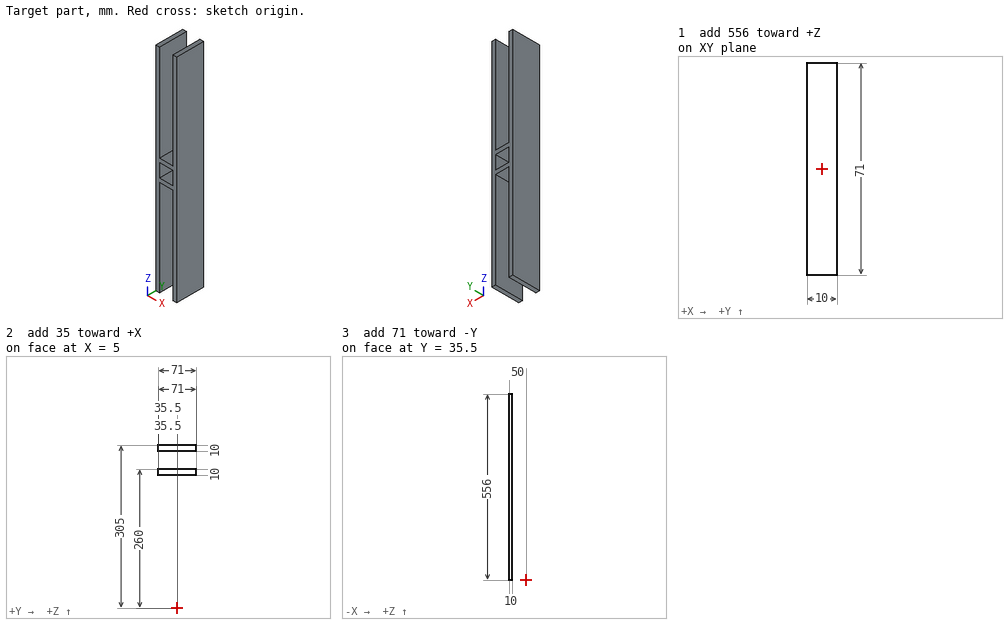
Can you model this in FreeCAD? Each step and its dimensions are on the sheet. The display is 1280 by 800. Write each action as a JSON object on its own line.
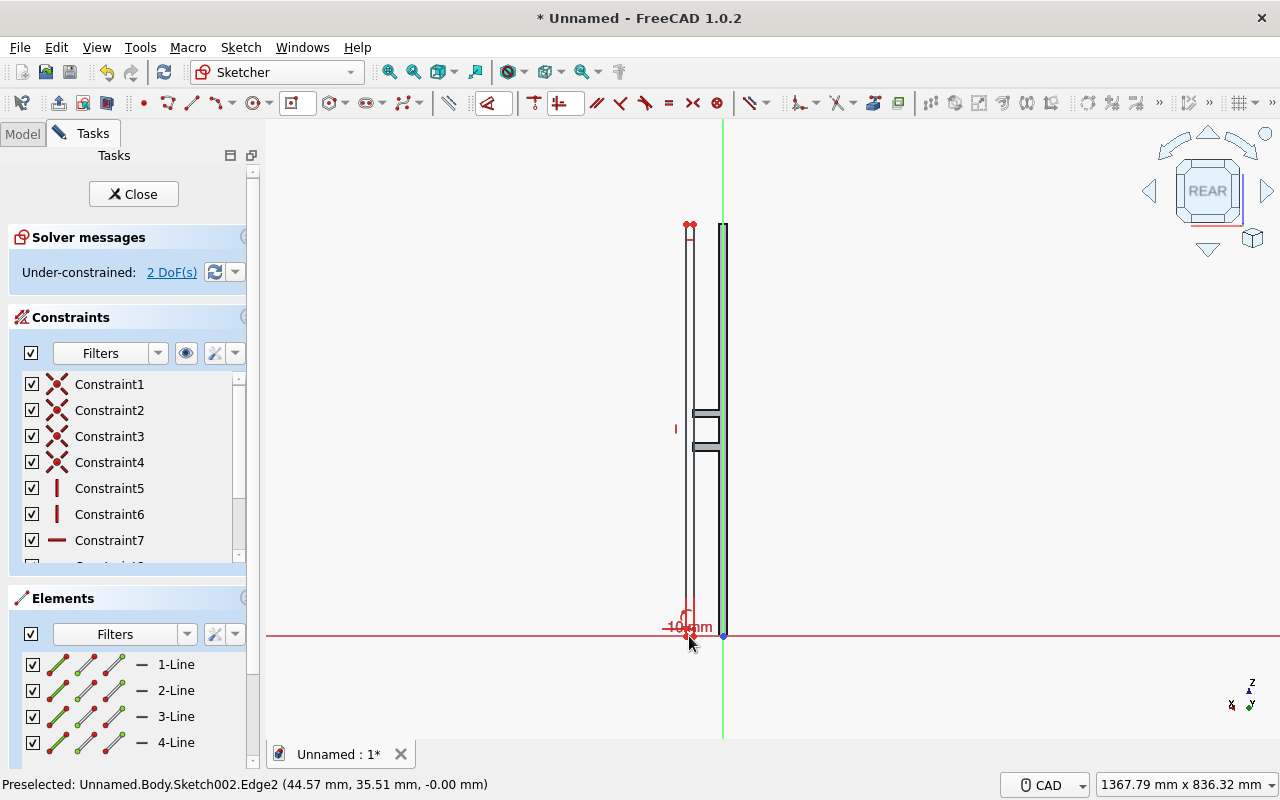
{"action": "scroll", "coordinate": [686, 348], "scroll_direction": "up", "scroll_amount": 4}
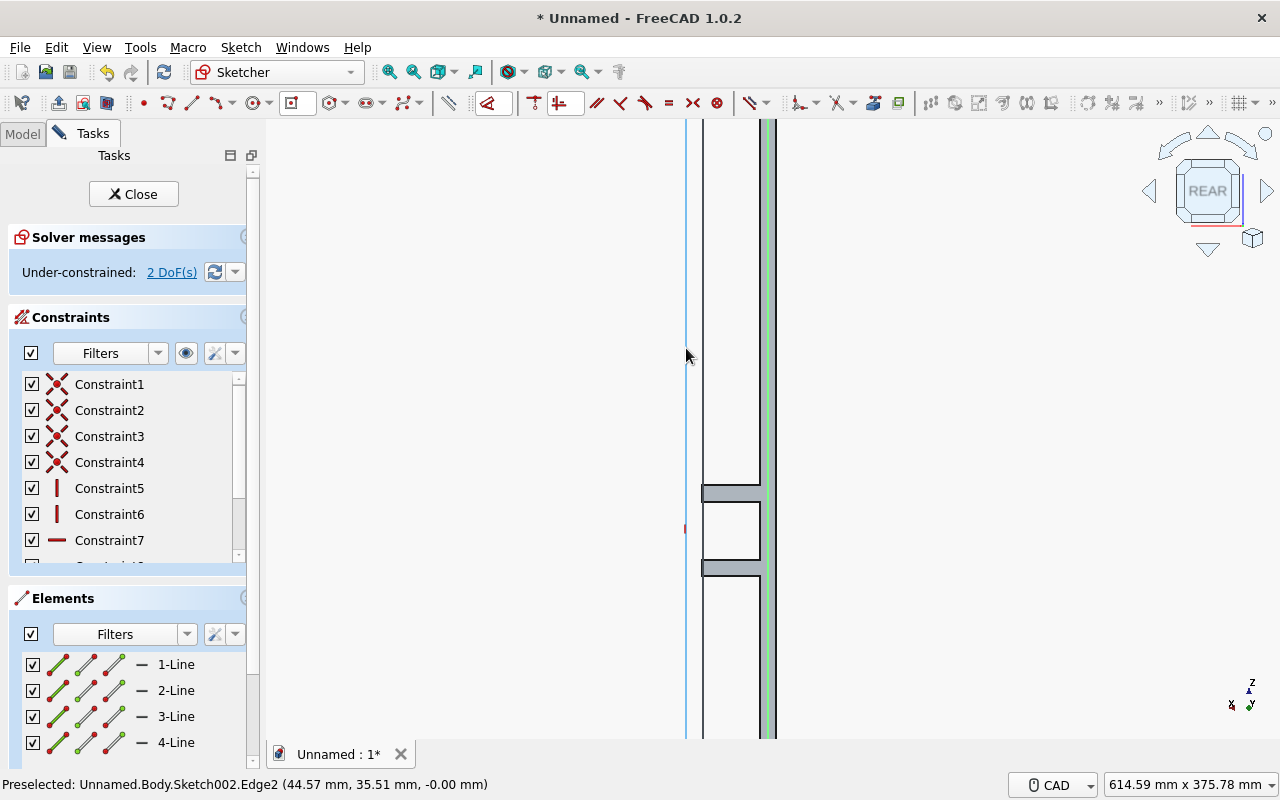
{"action": "left_click", "coordinate": [686, 347]}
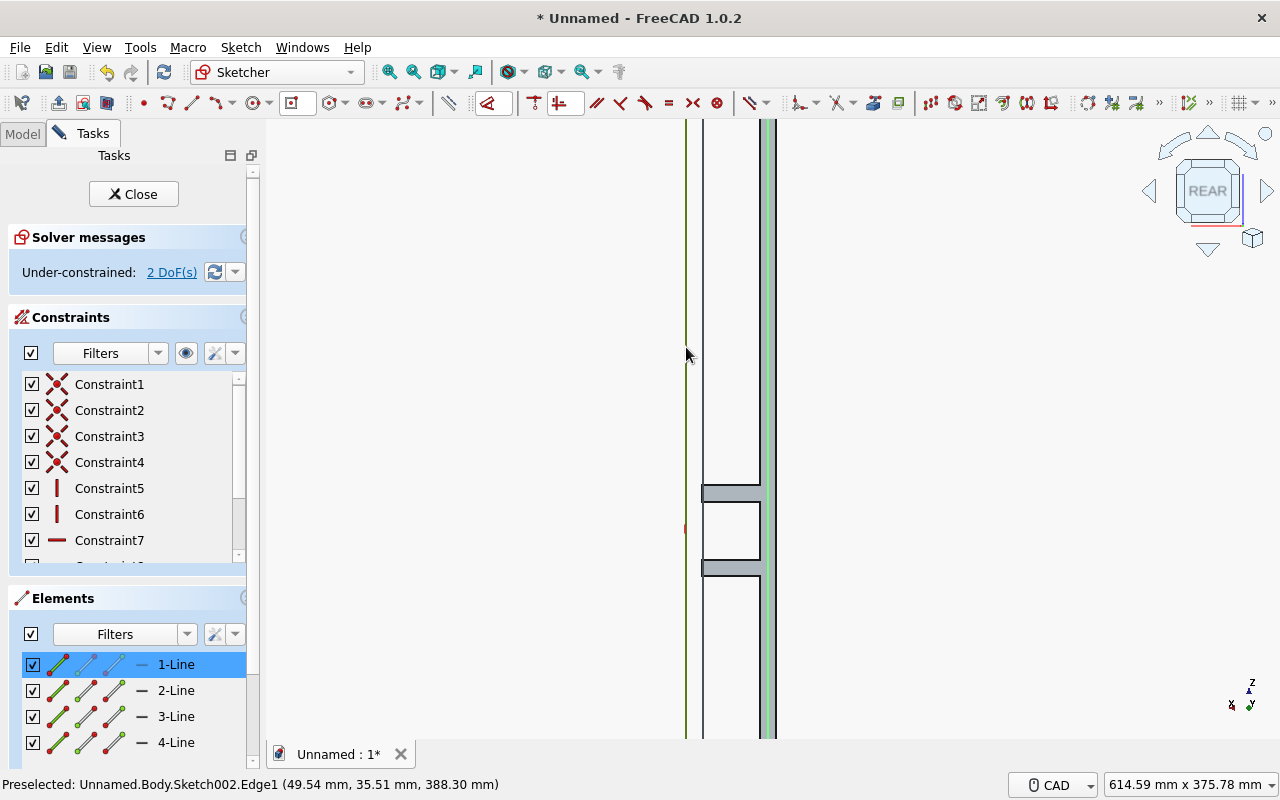
{"action": "key", "text": "i"}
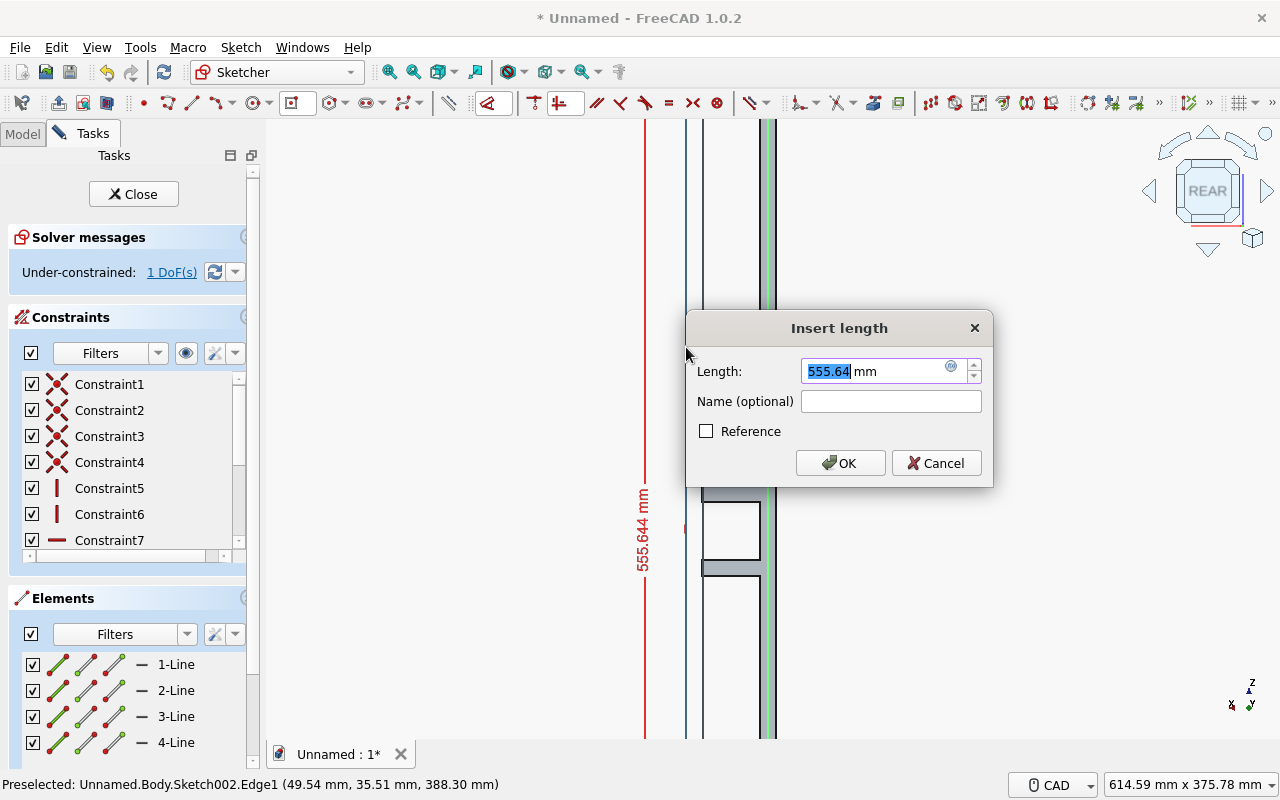
{"action": "type", "text": "556"}
{"action": "key", "text": "Return"}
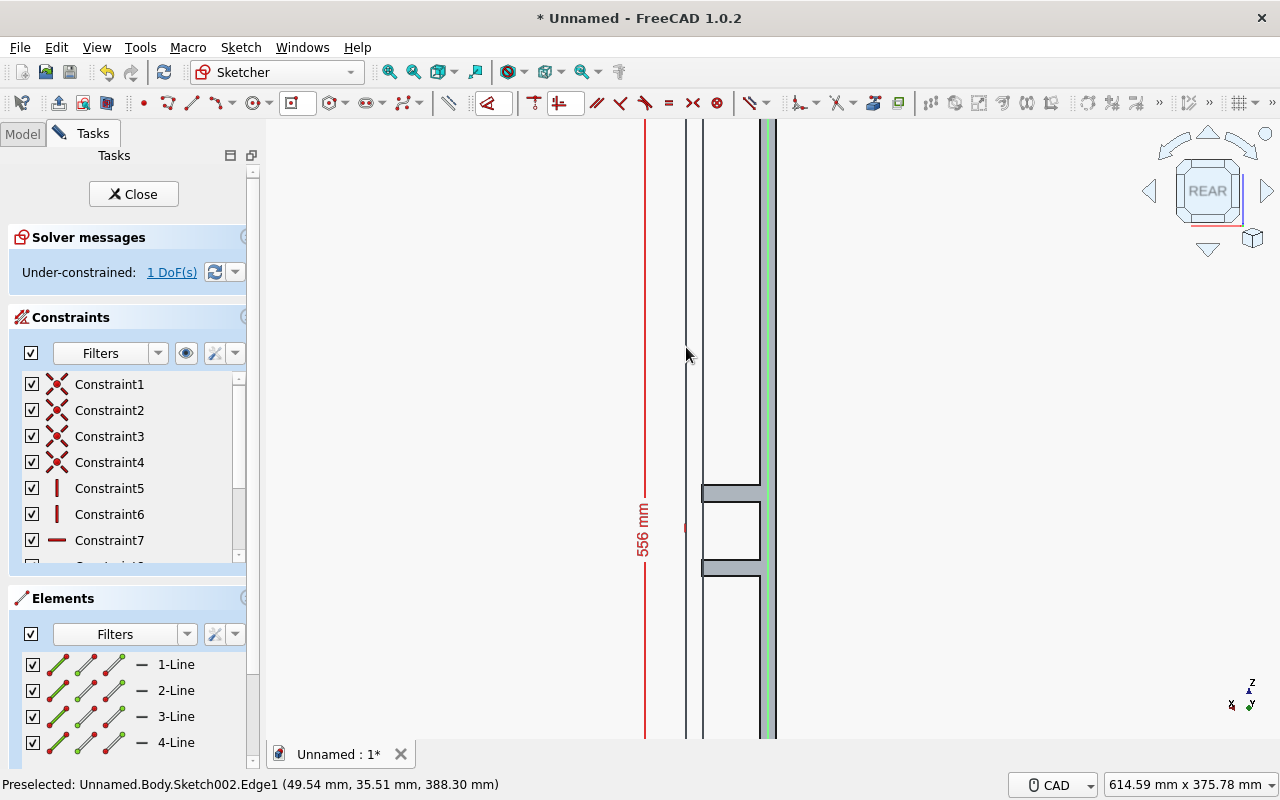
{"action": "scroll", "coordinate": [686, 347], "scroll_direction": "down", "scroll_amount": 4}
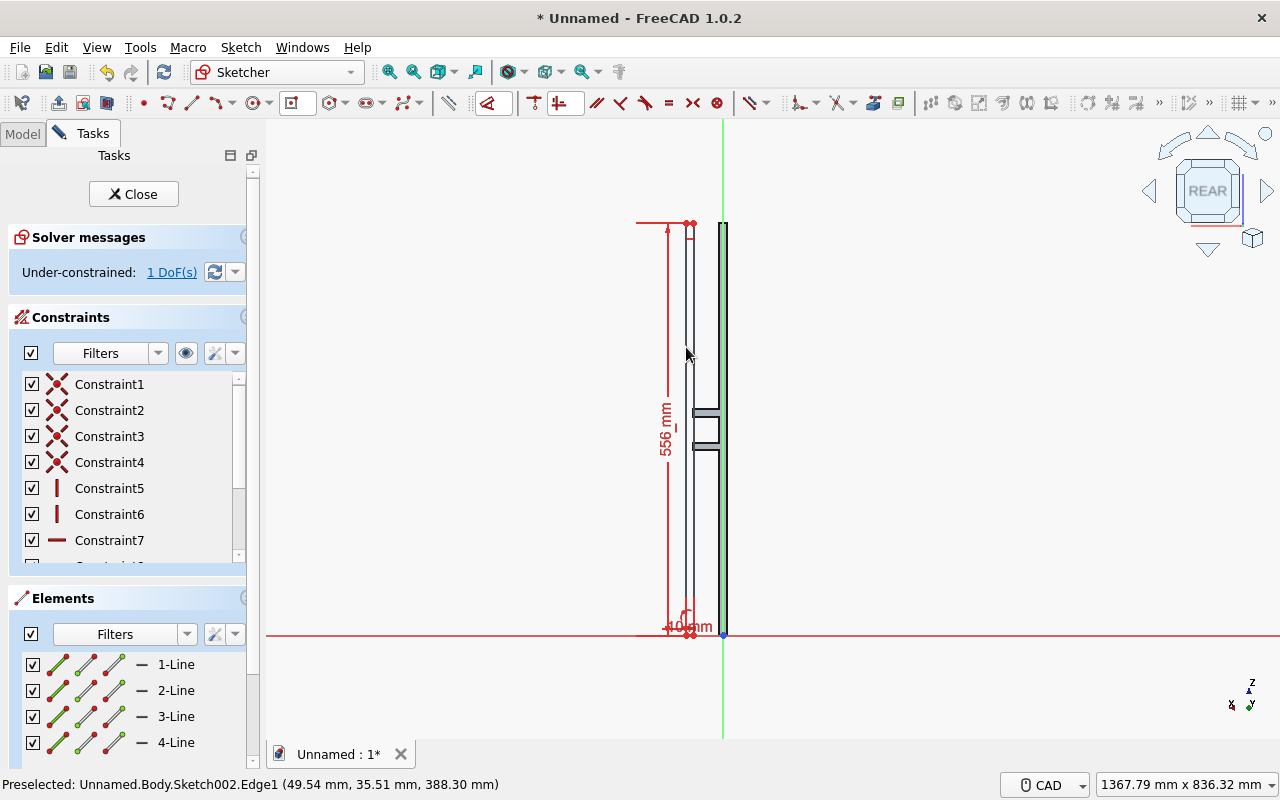
{"action": "scroll", "coordinate": [686, 223], "scroll_direction": "up", "scroll_amount": 3}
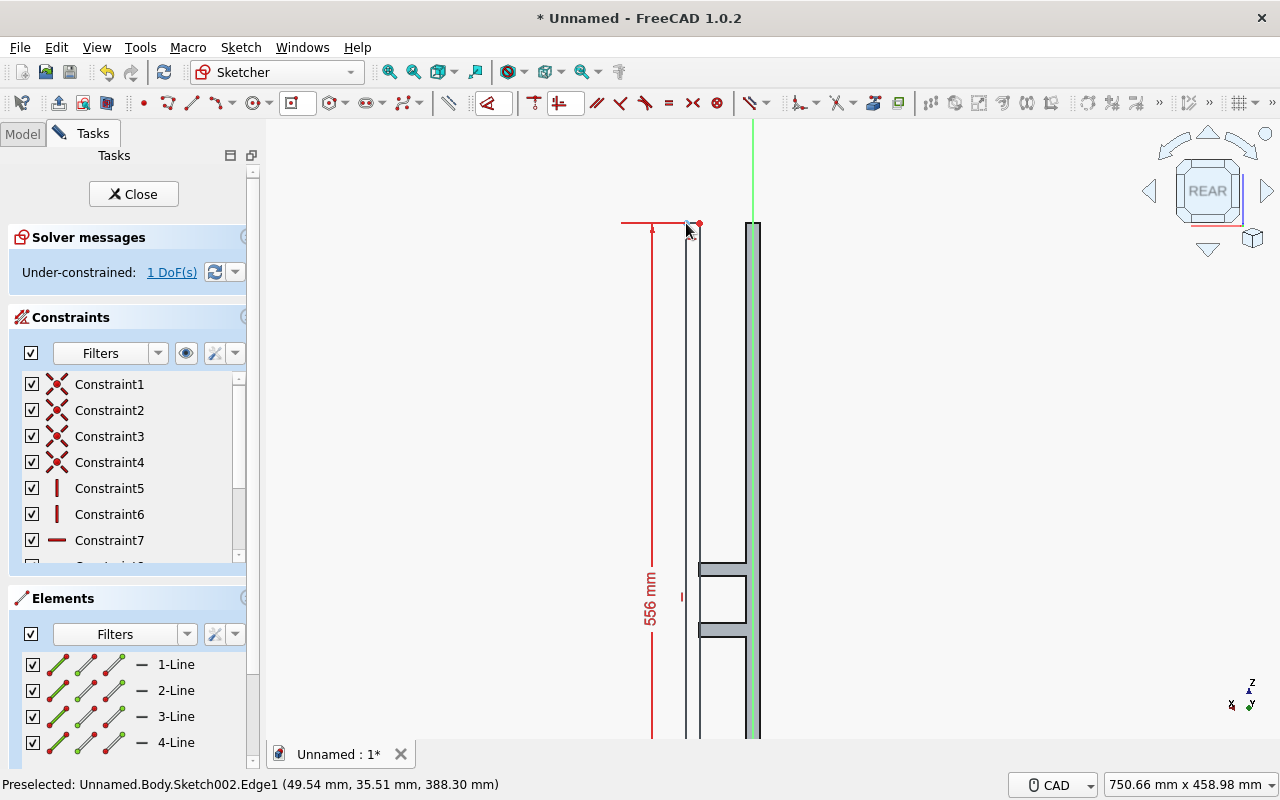
{"action": "left_click", "coordinate": [686, 223]}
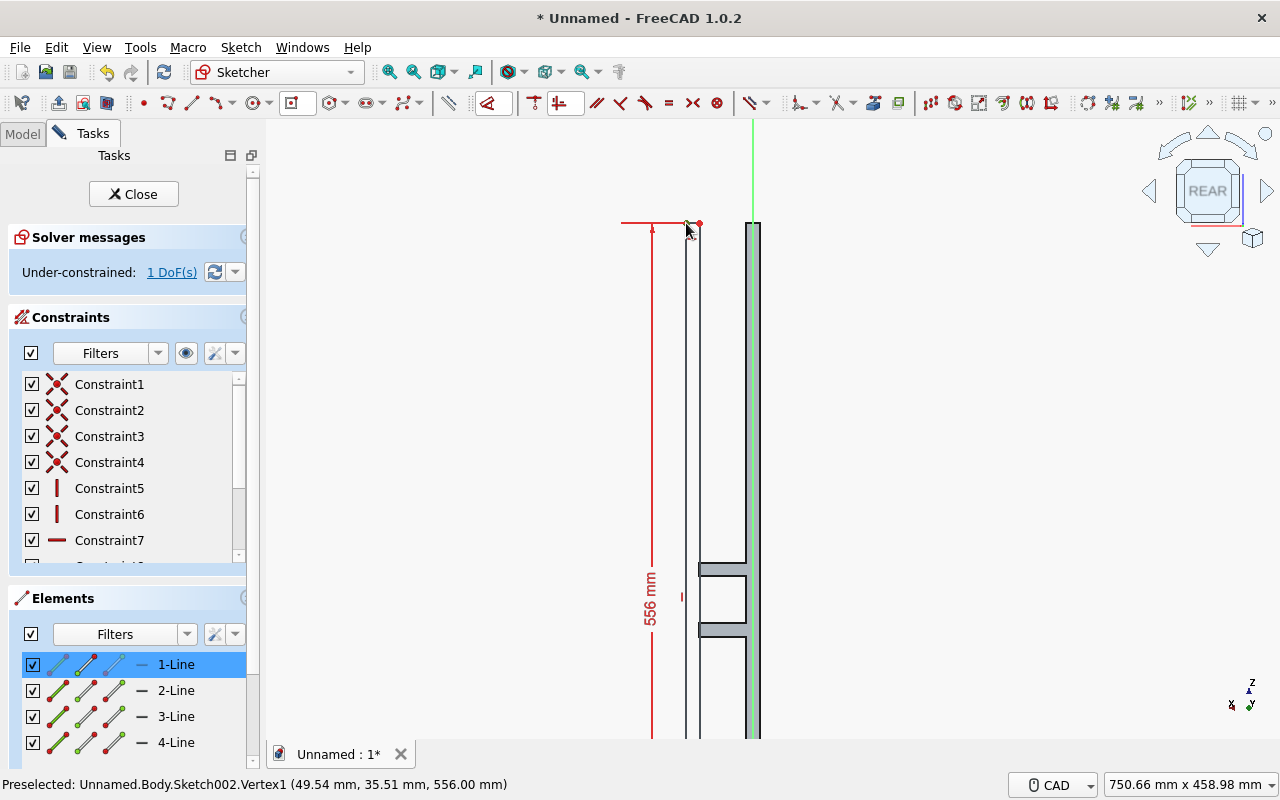
{"action": "key", "text": "l"}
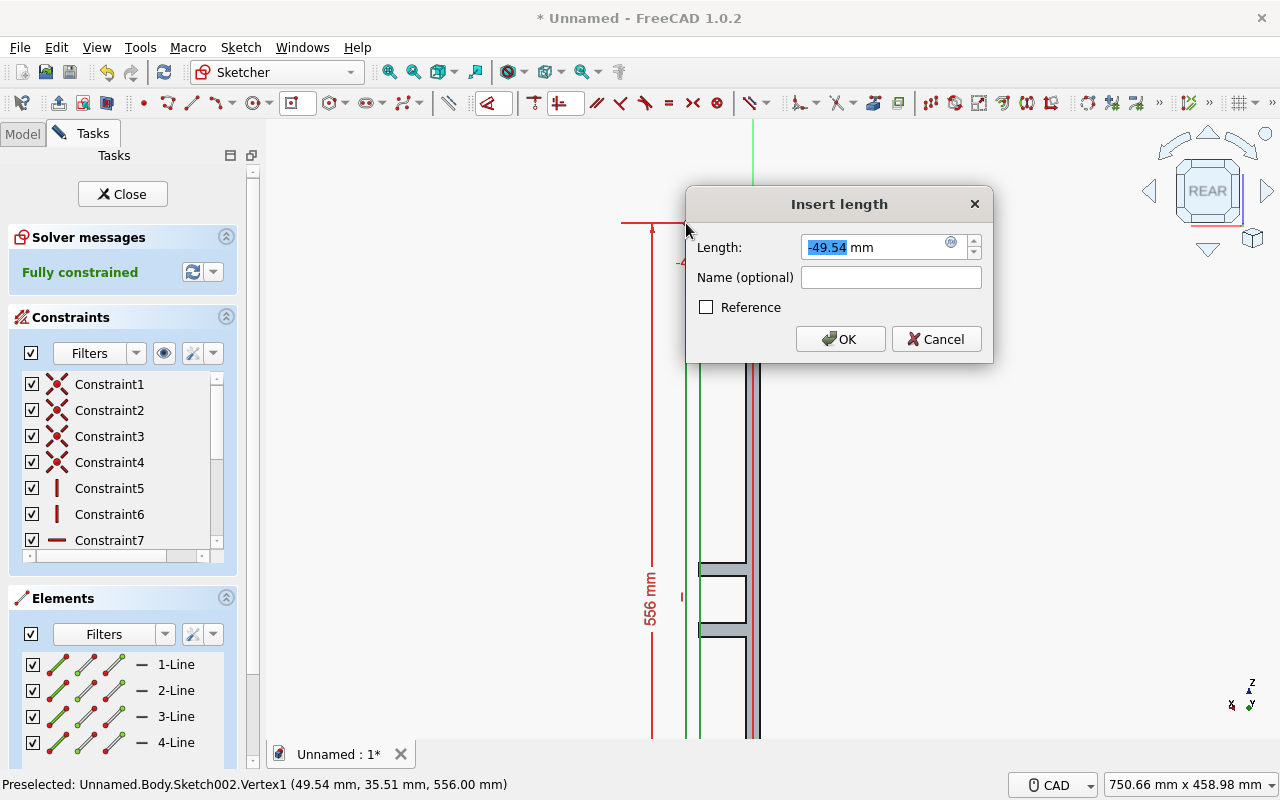
{"action": "type", "text": "-50"}
{"action": "key", "text": "Return"}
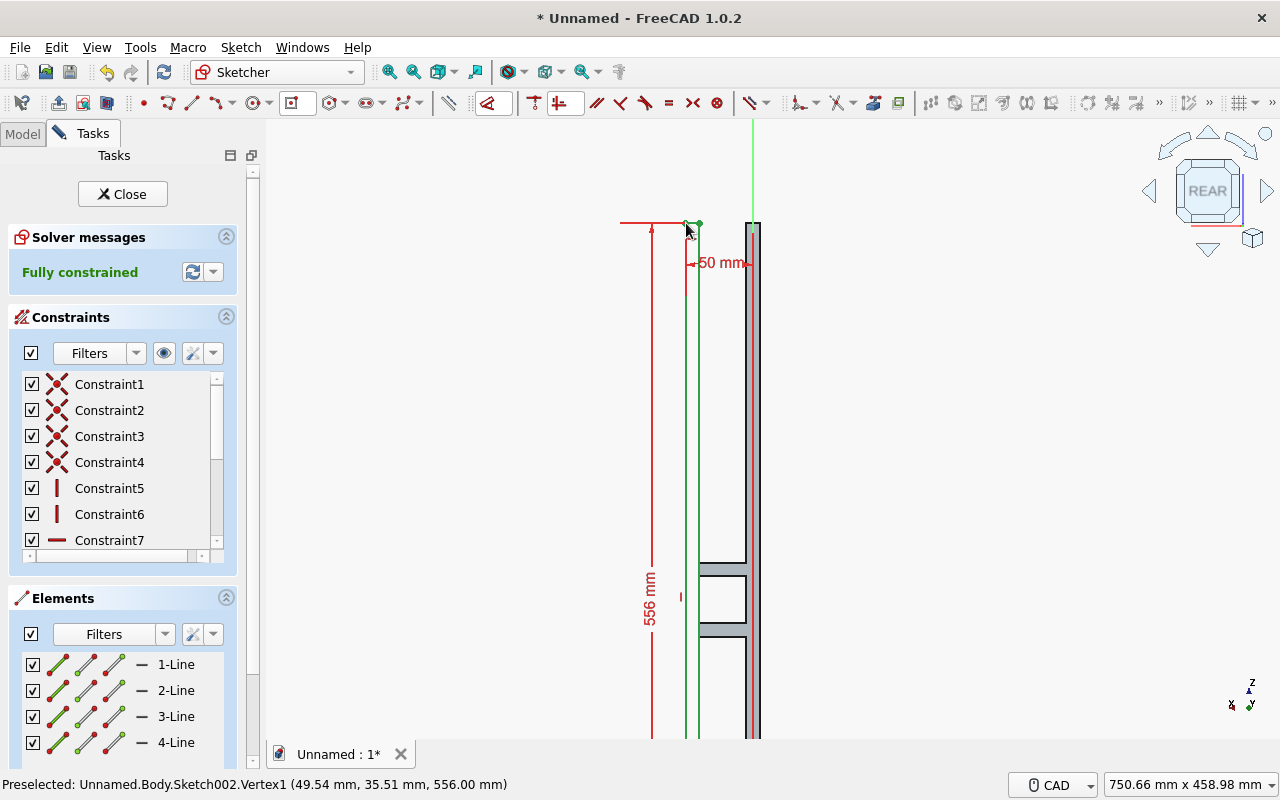
{"action": "left_click", "coordinate": [123, 194]}